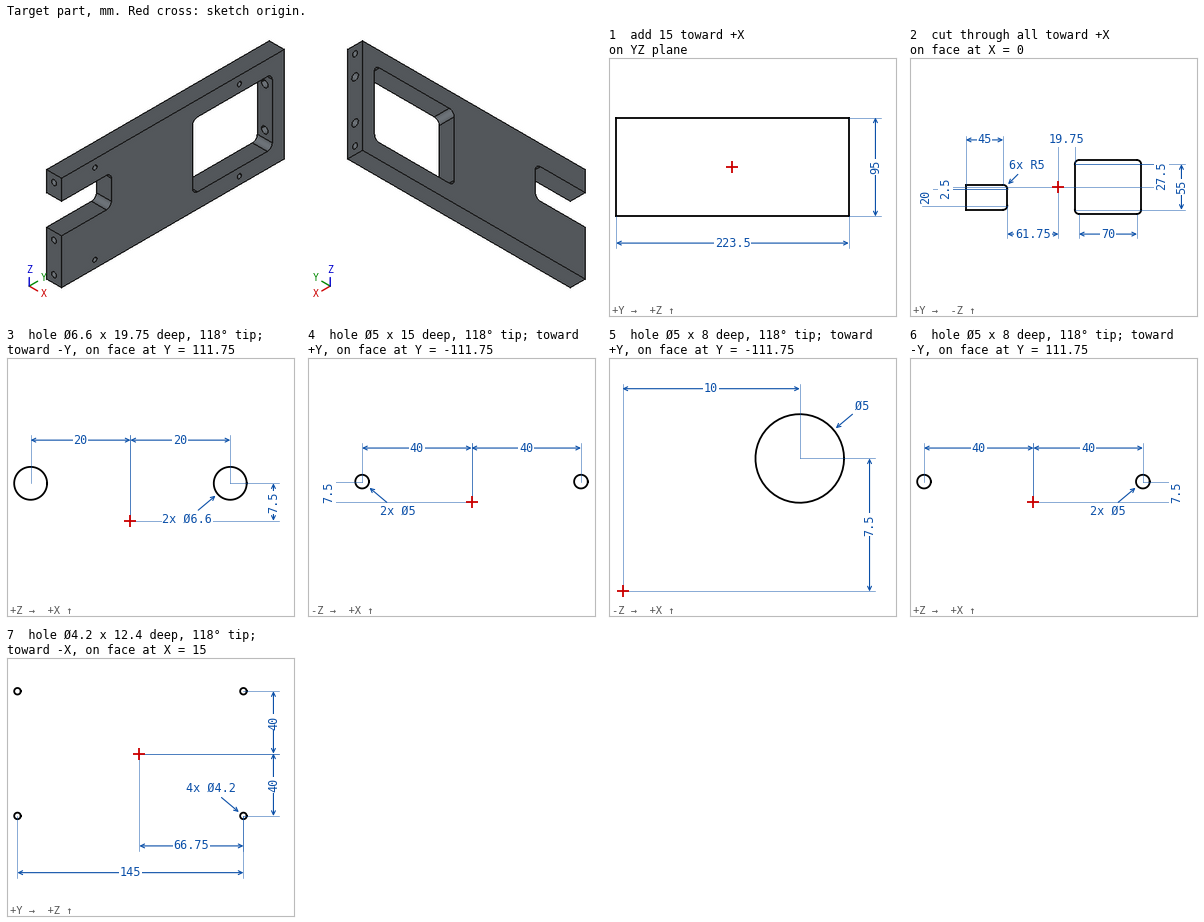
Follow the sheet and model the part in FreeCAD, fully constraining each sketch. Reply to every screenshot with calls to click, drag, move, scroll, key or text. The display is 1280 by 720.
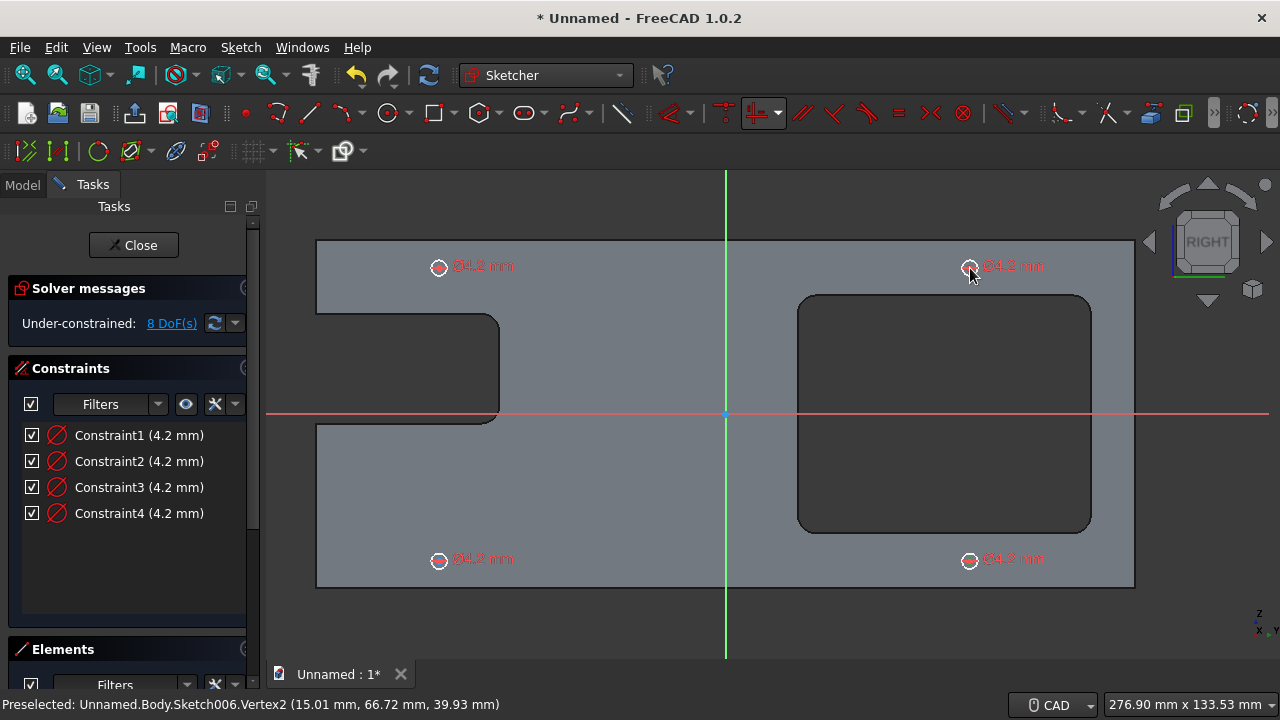
key(v)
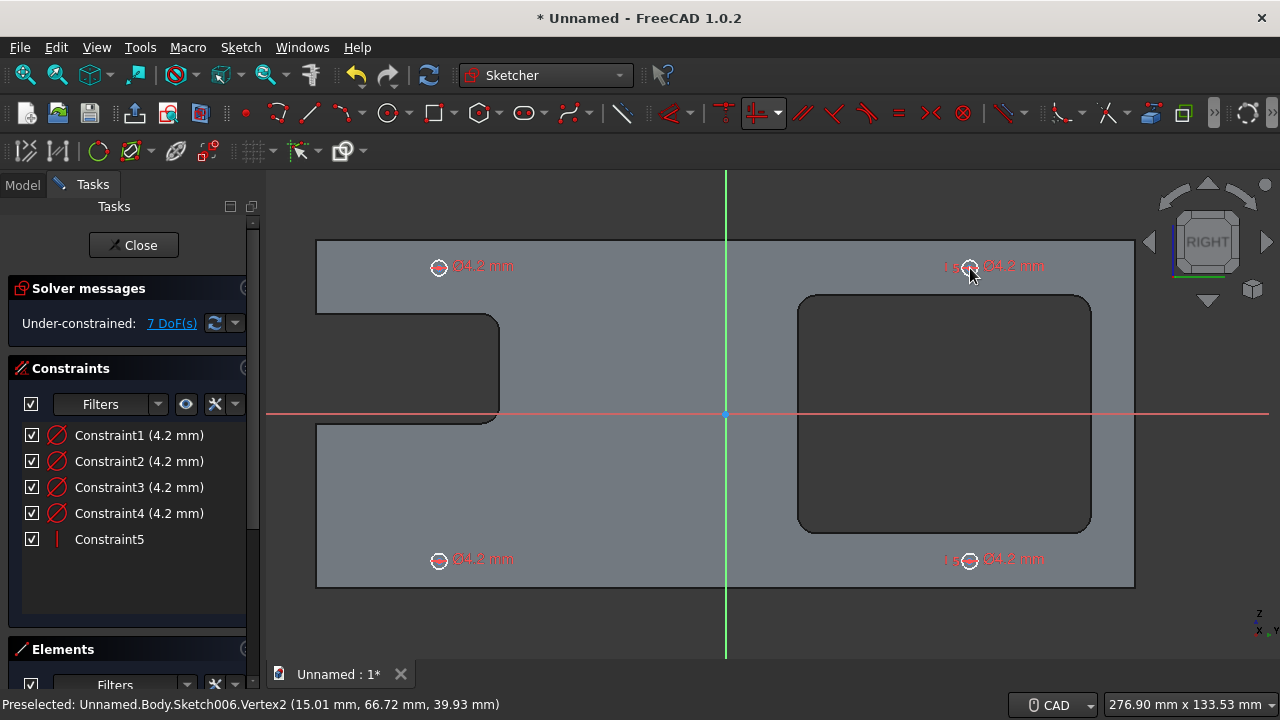
click(970, 561)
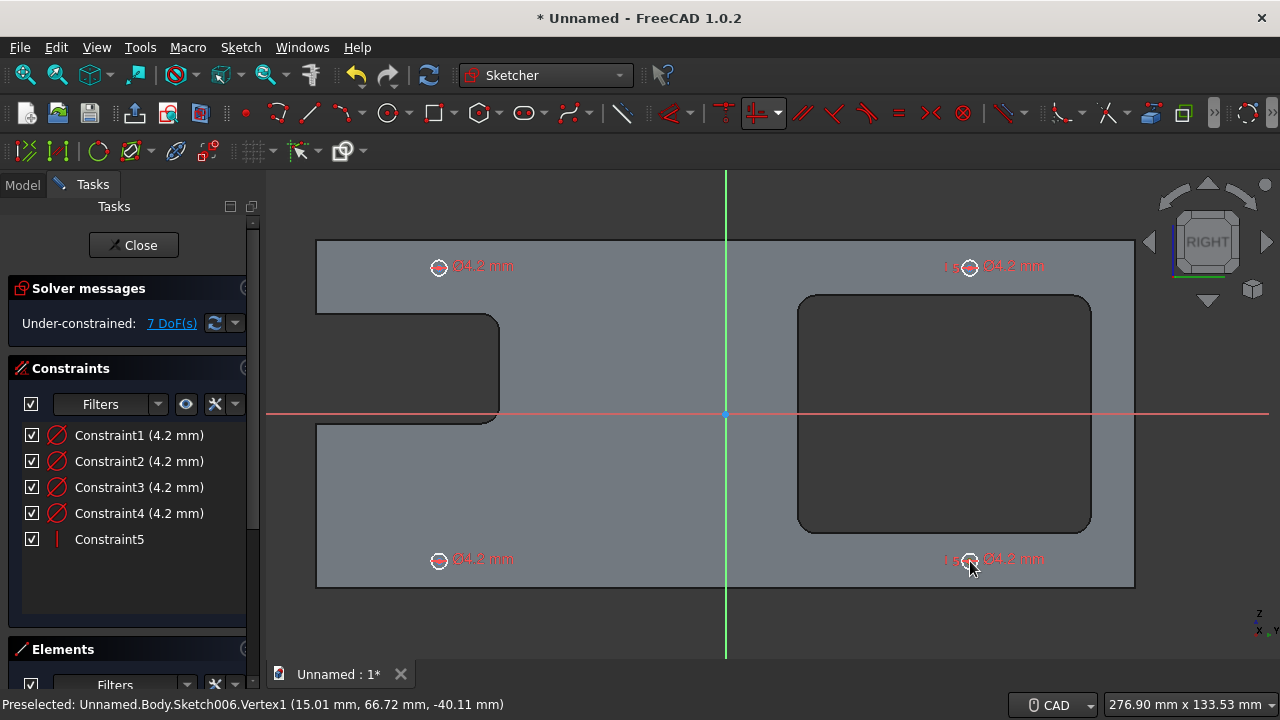
click(439, 561)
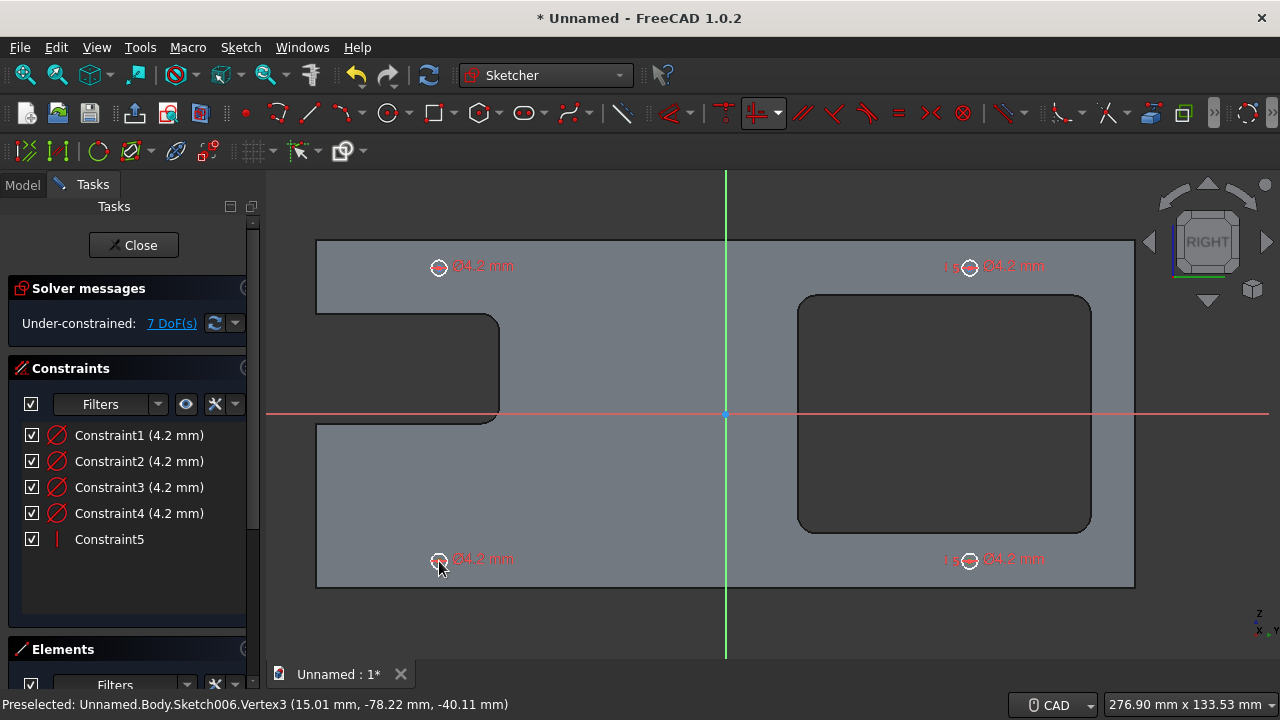
key(h)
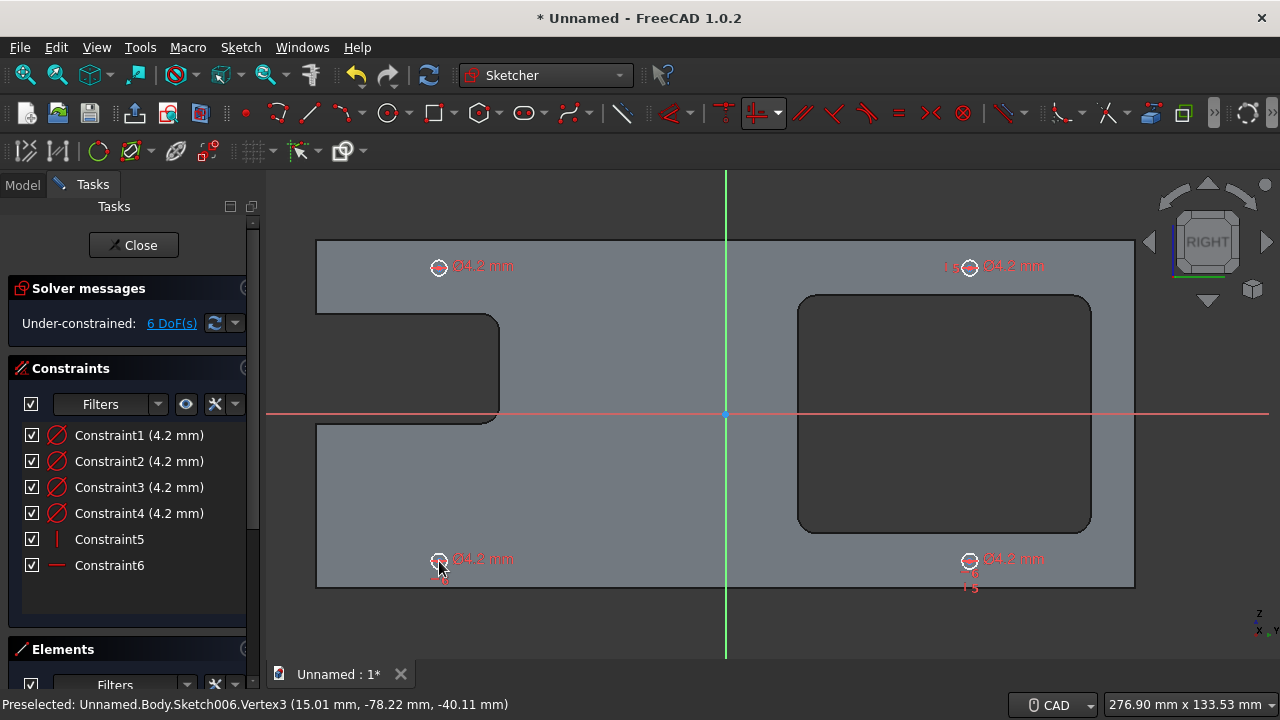
click(439, 561)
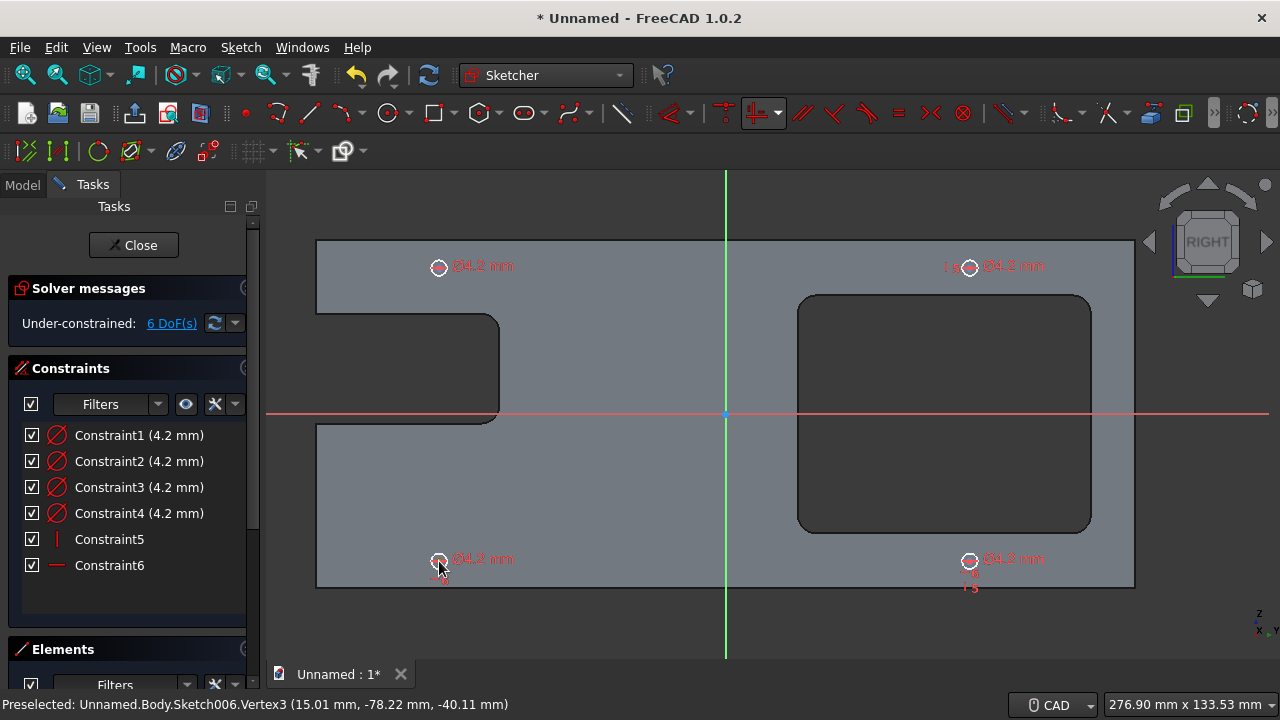
click(439, 268)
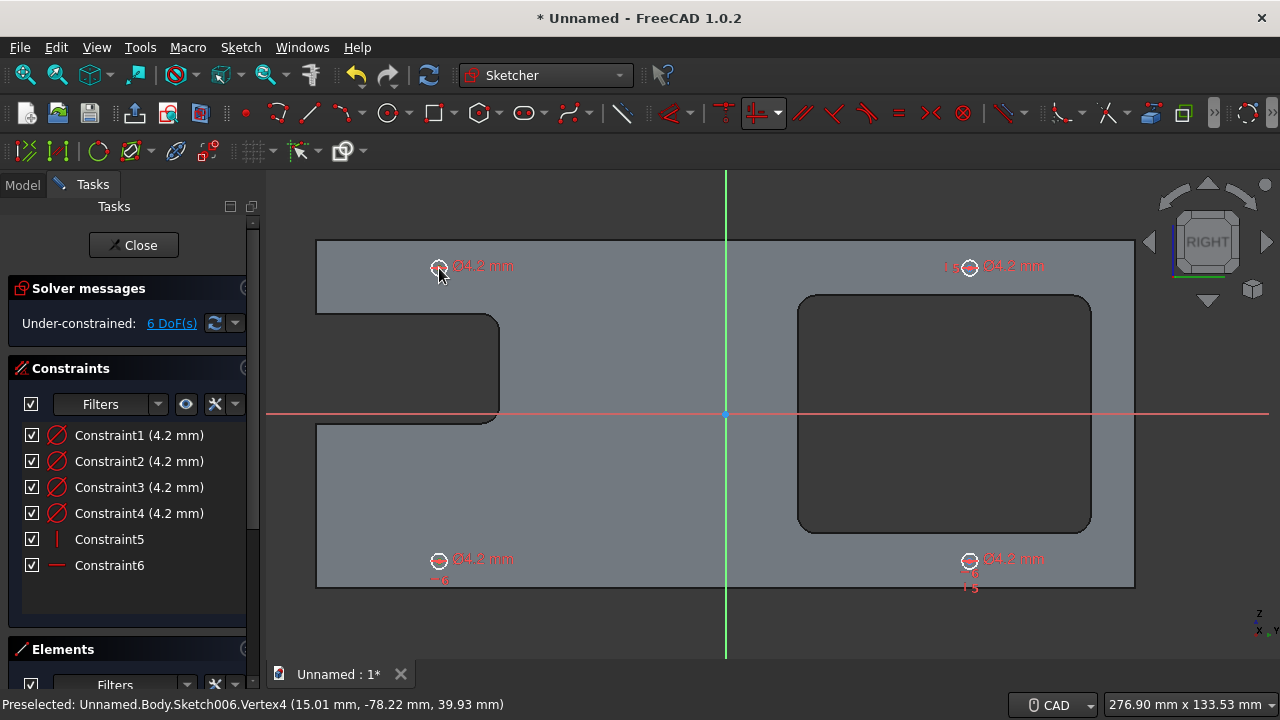
key(v)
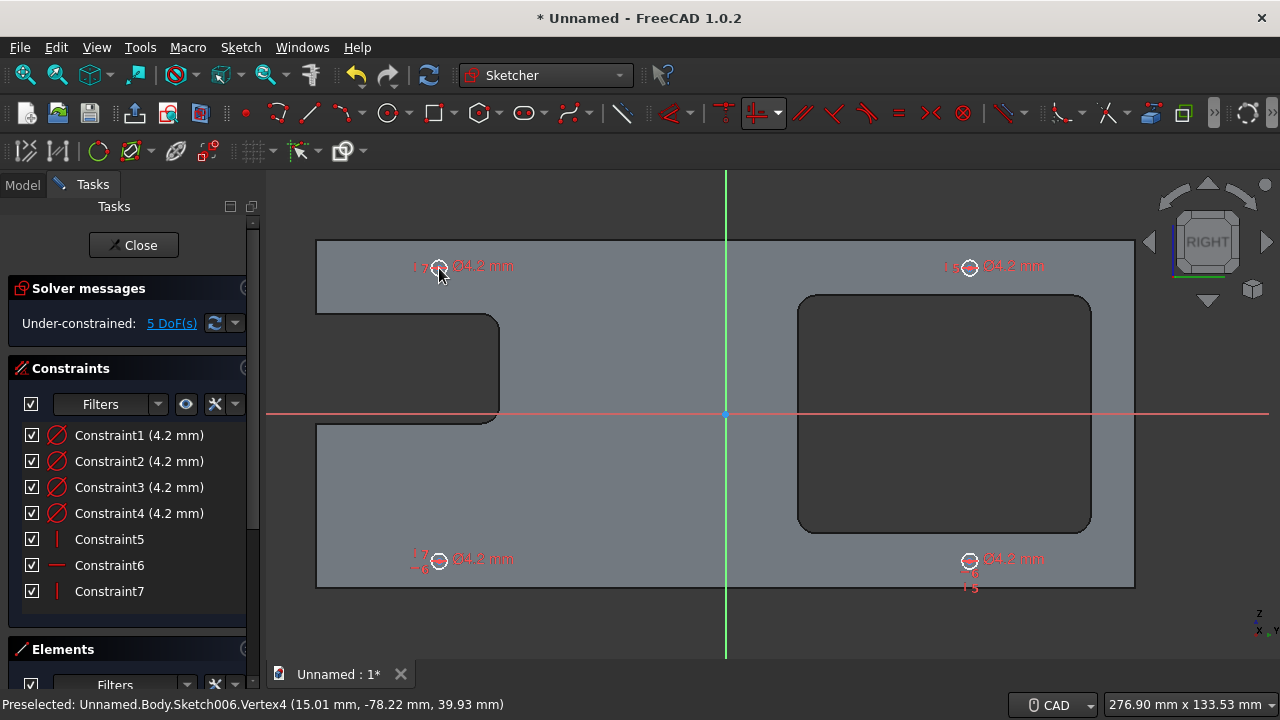
click(970, 268)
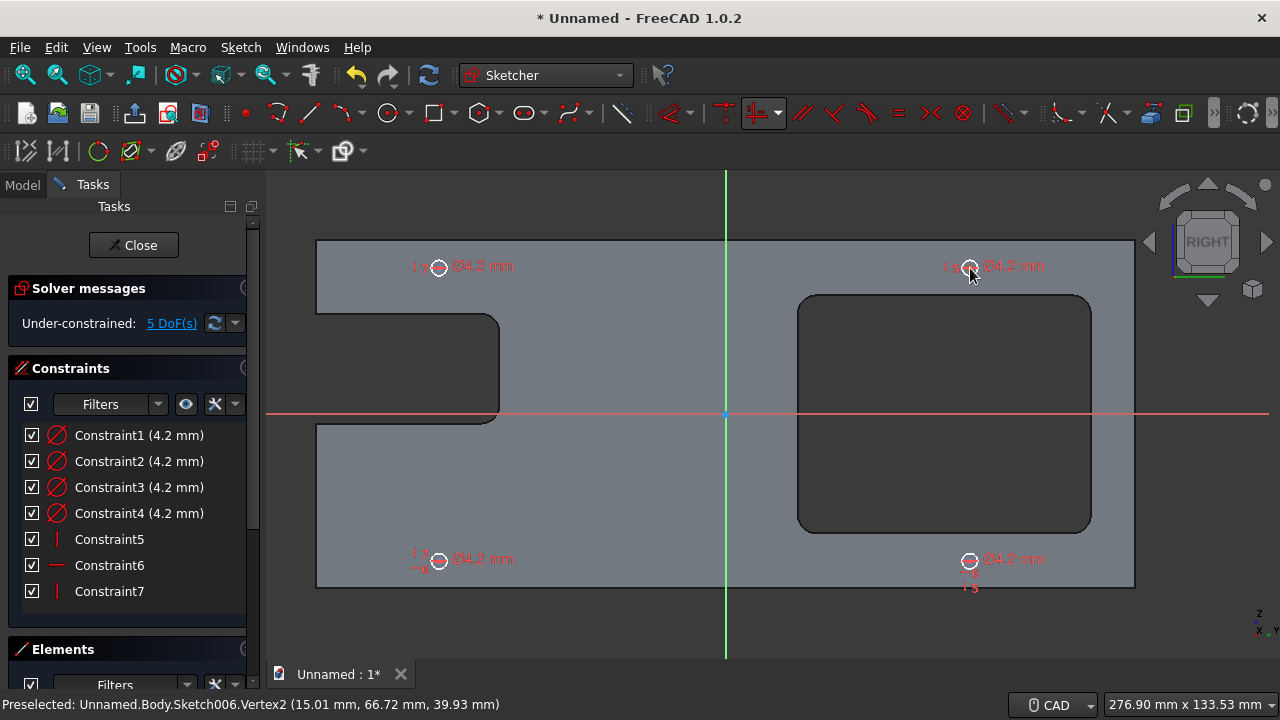
click(439, 268)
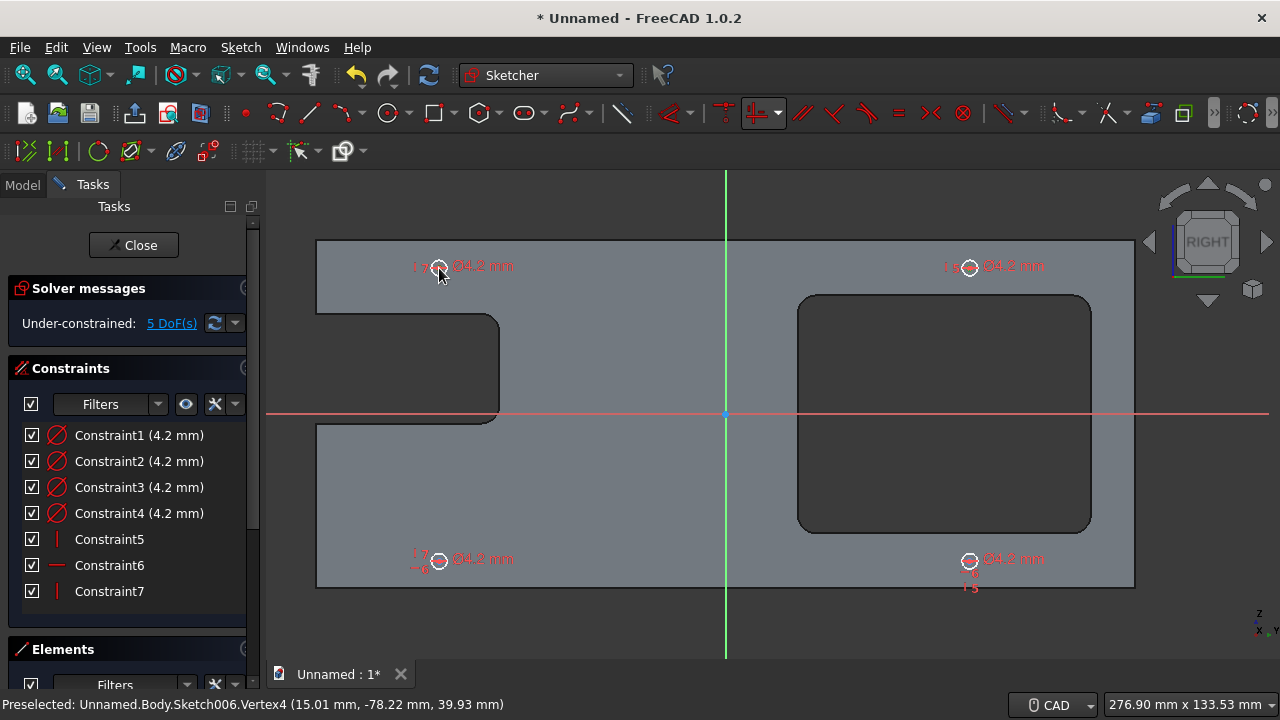
click(780, 114)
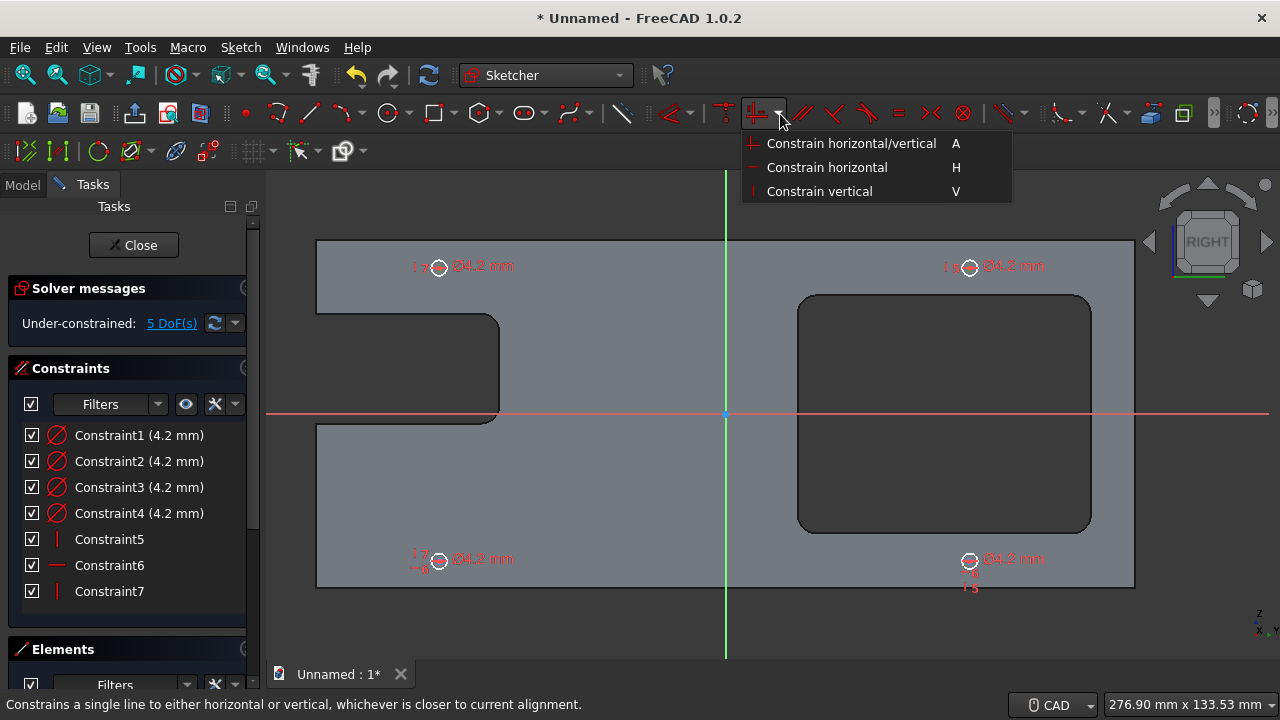
click(877, 167)